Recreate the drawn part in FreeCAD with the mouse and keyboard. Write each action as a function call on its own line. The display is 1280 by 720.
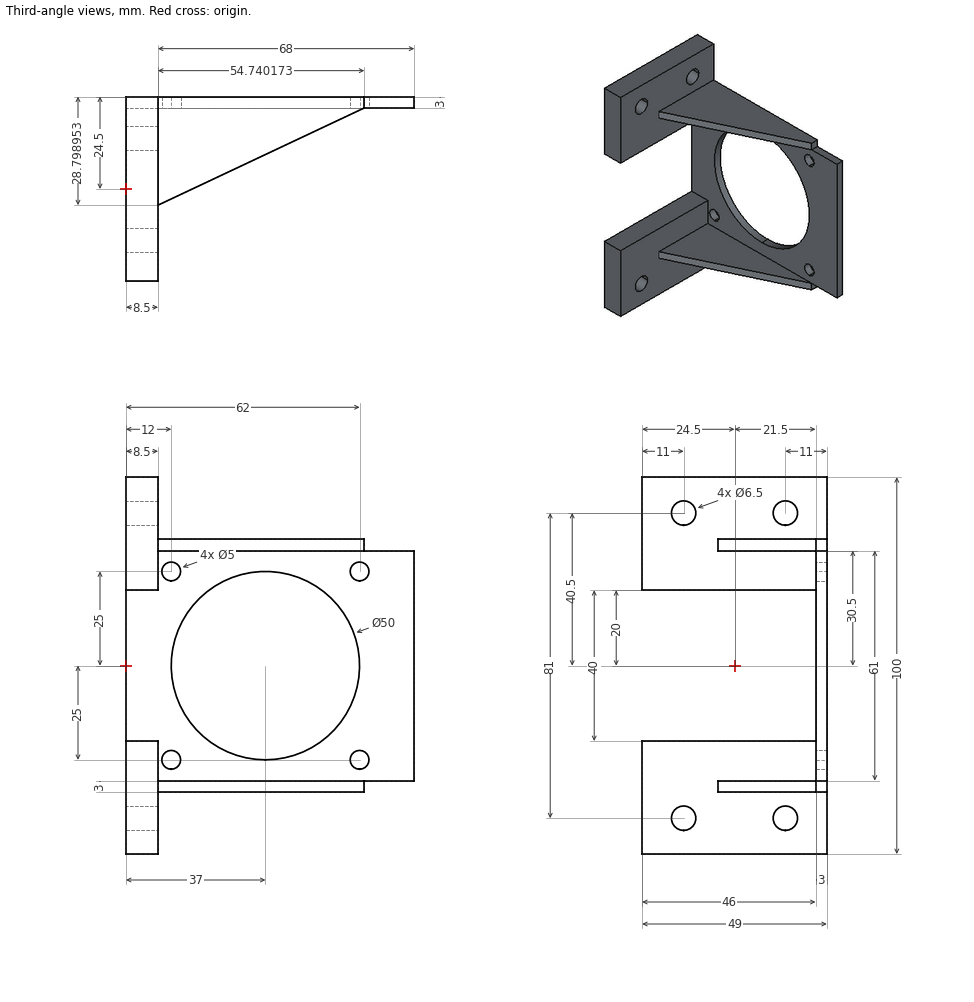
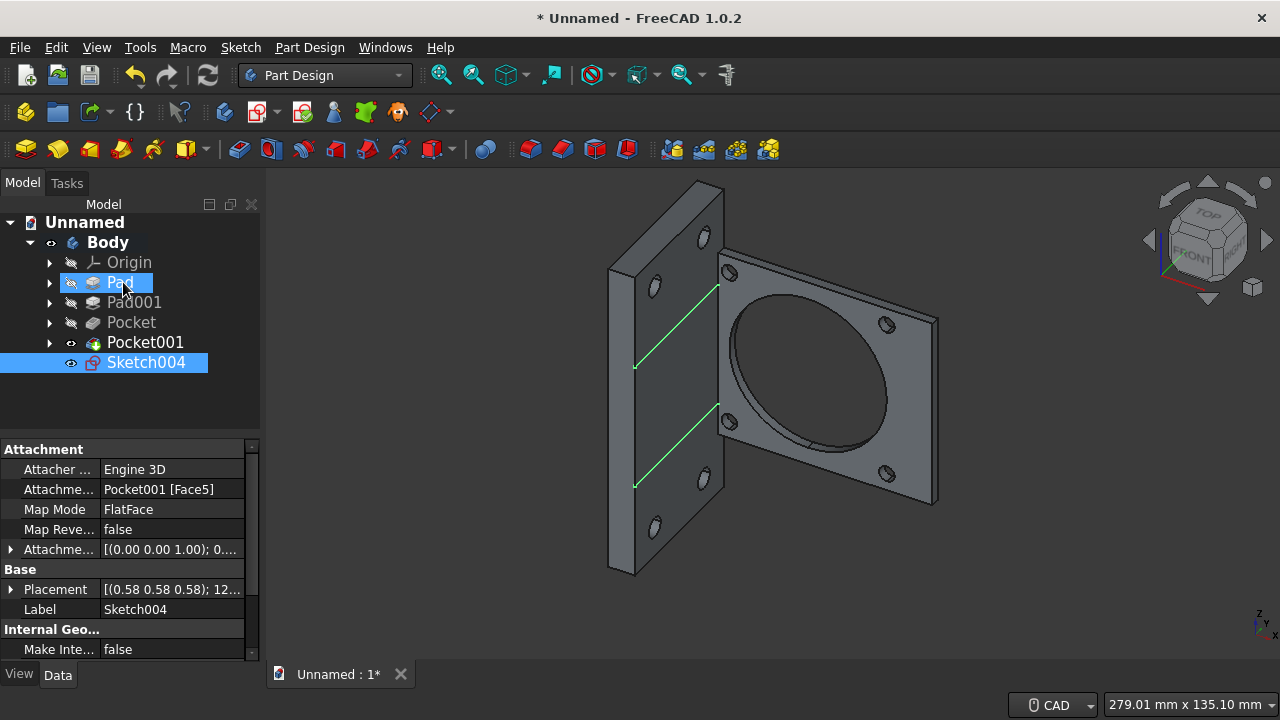
click(240, 150)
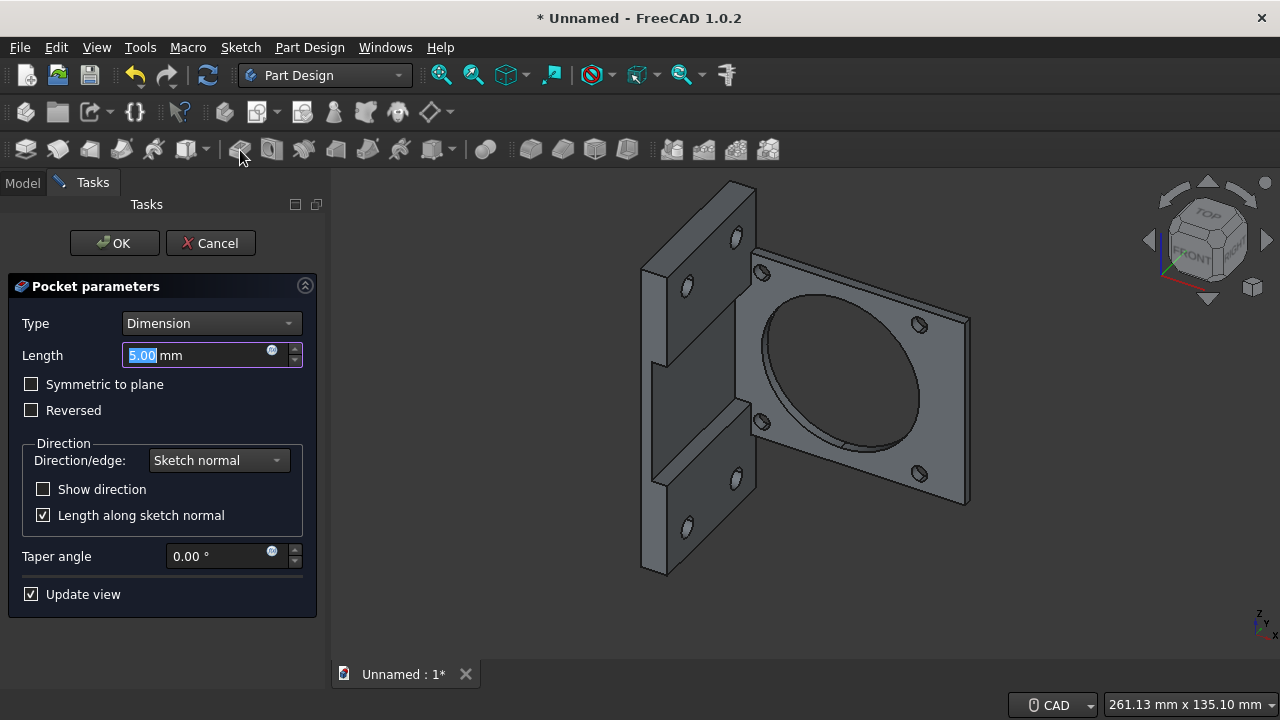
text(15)
key(Tab)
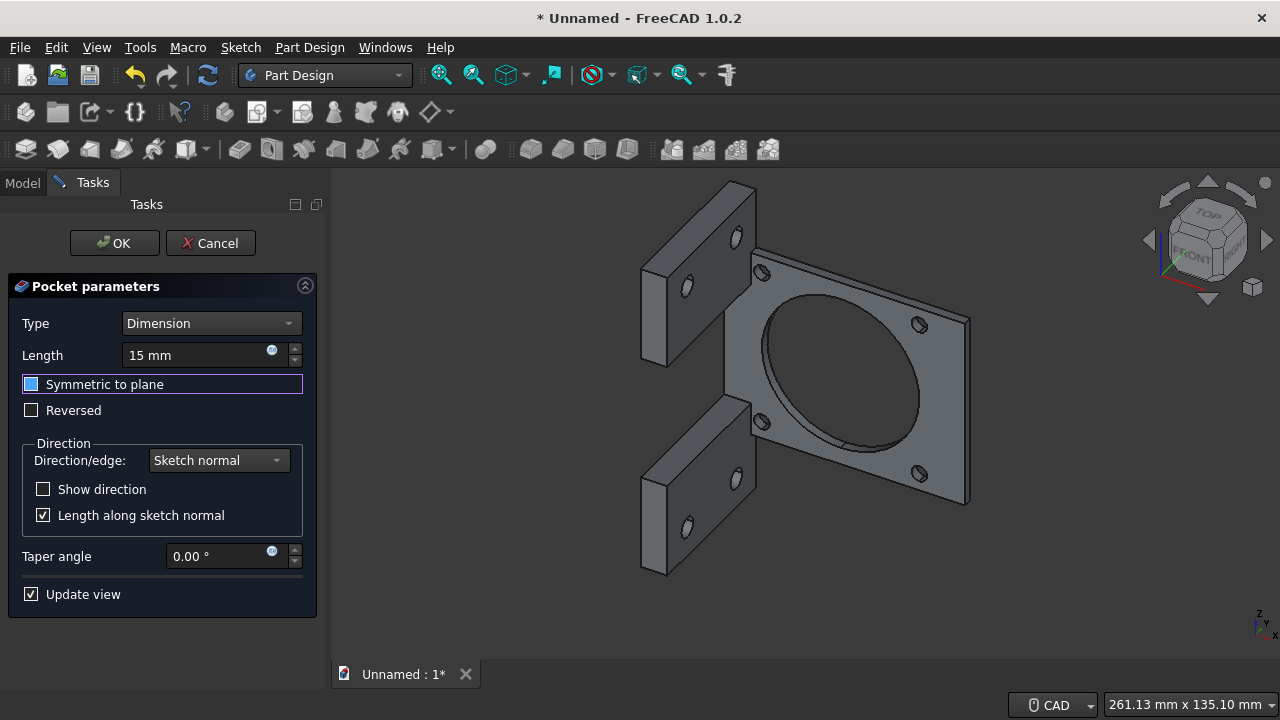
click(115, 243)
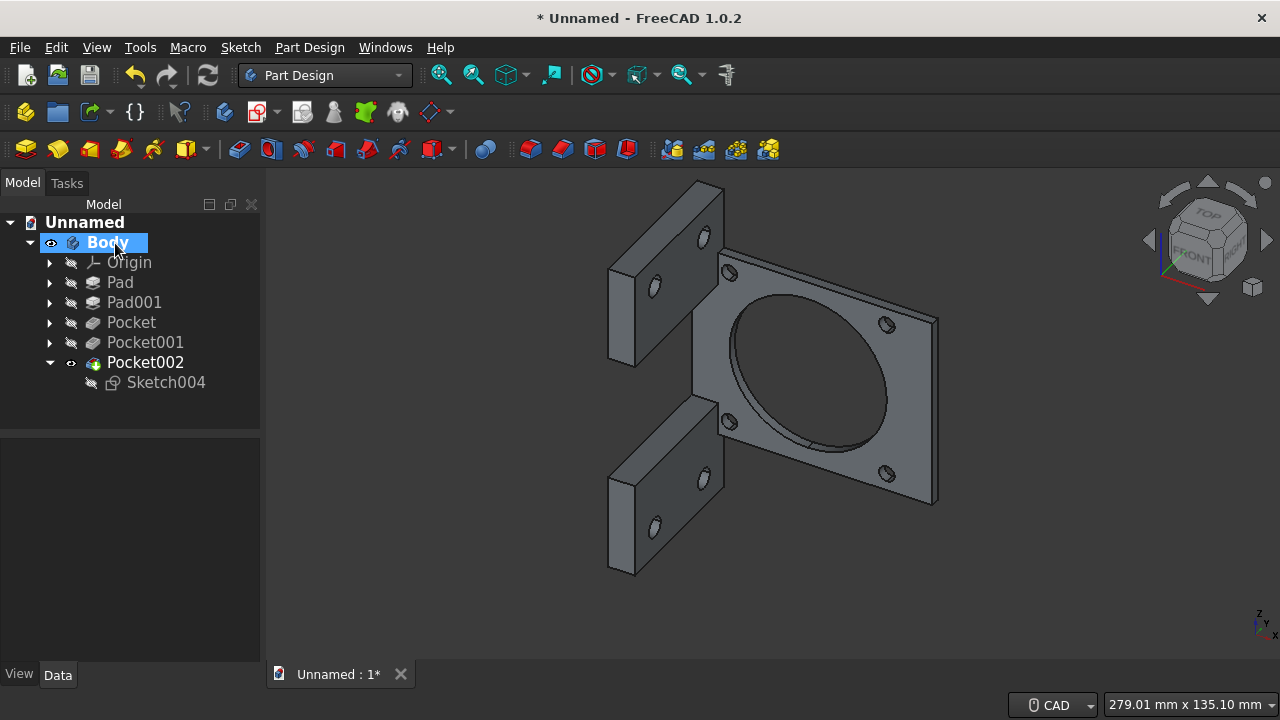
key(5)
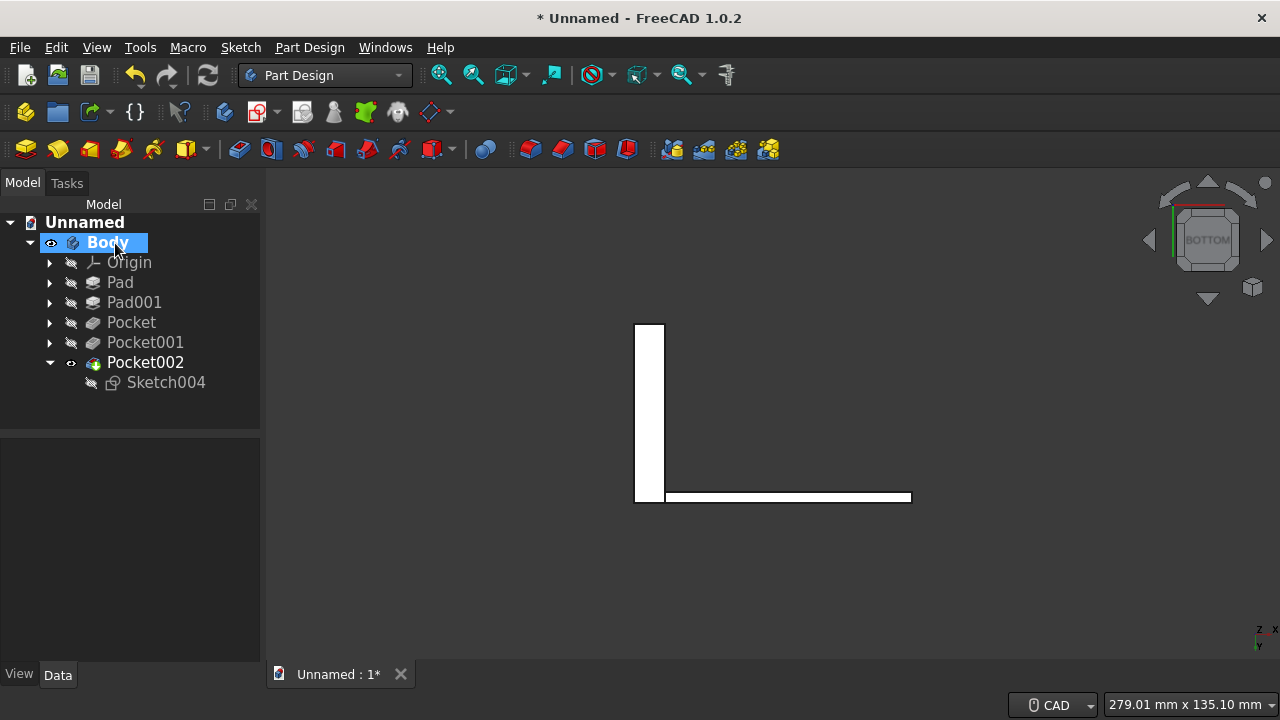
click(442, 76)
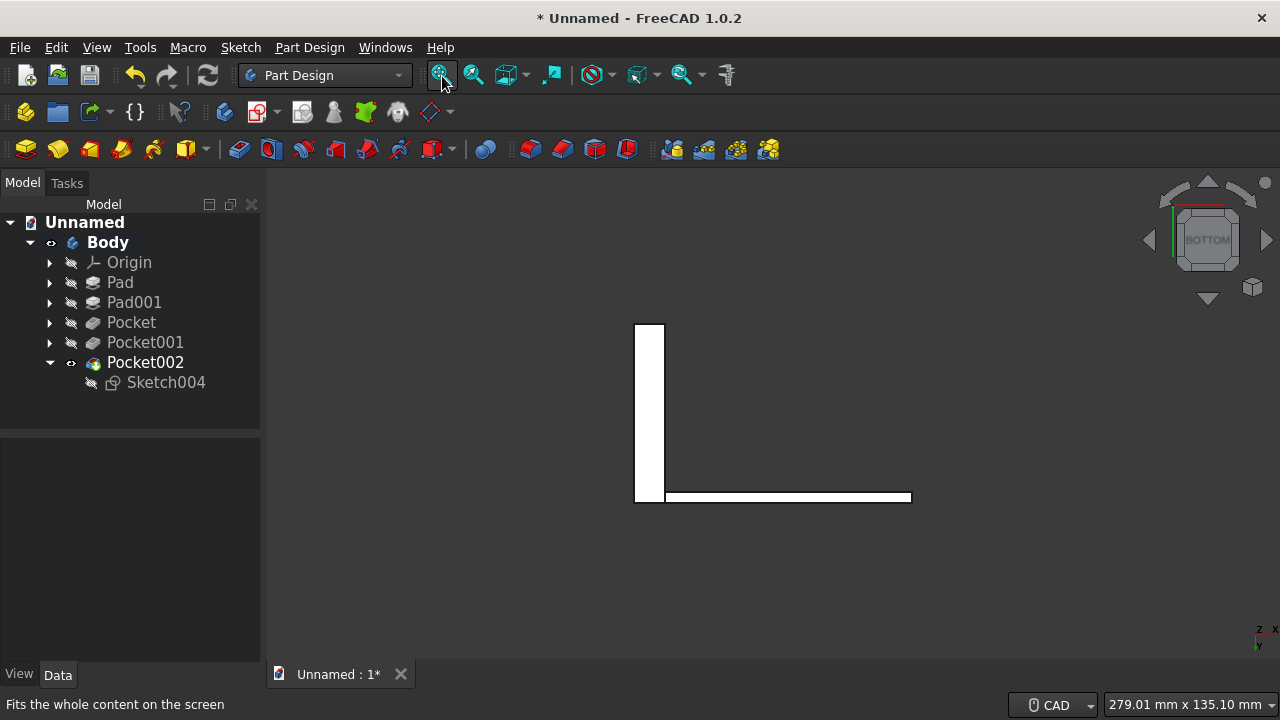
scroll(859, 496, up, 4)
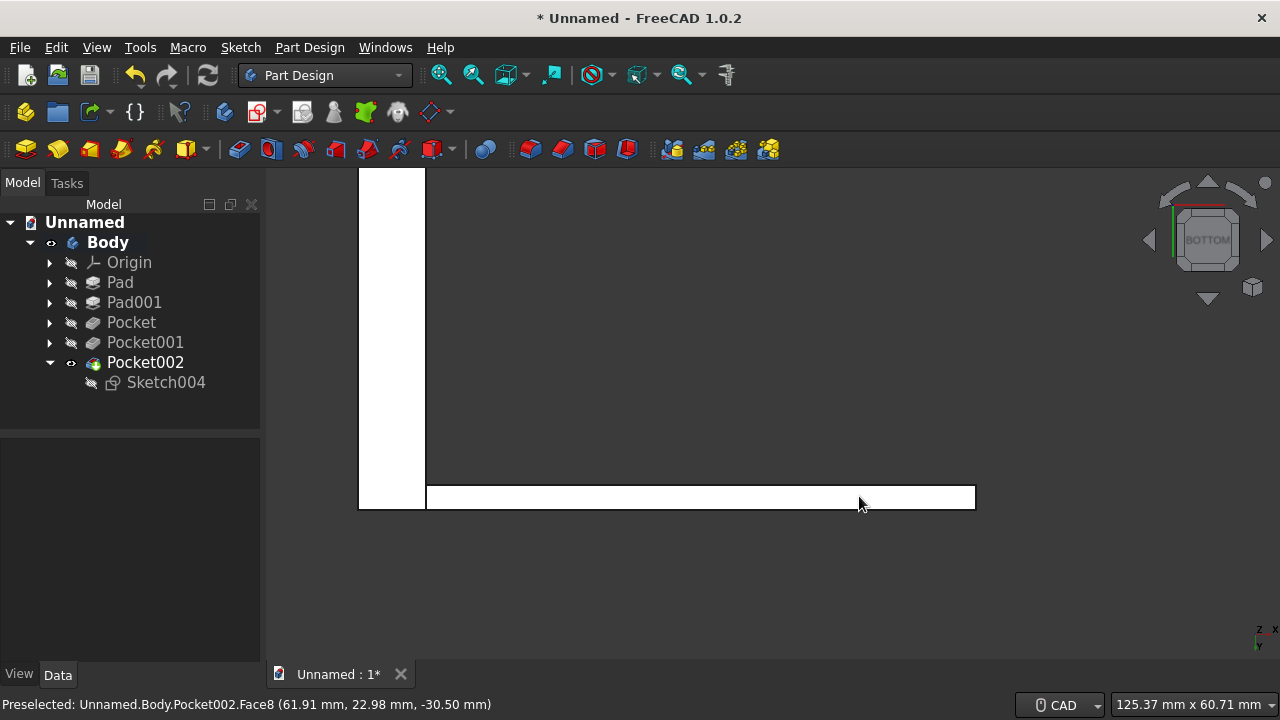
click(858, 497)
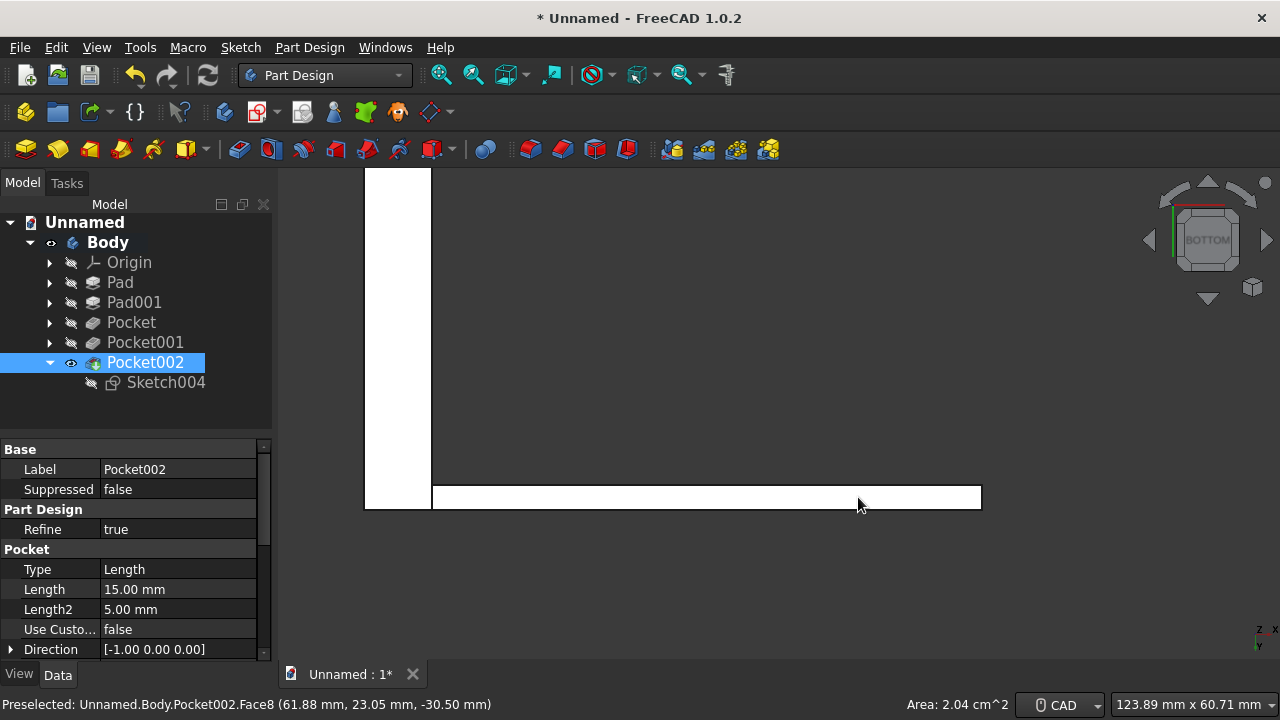
click(258, 112)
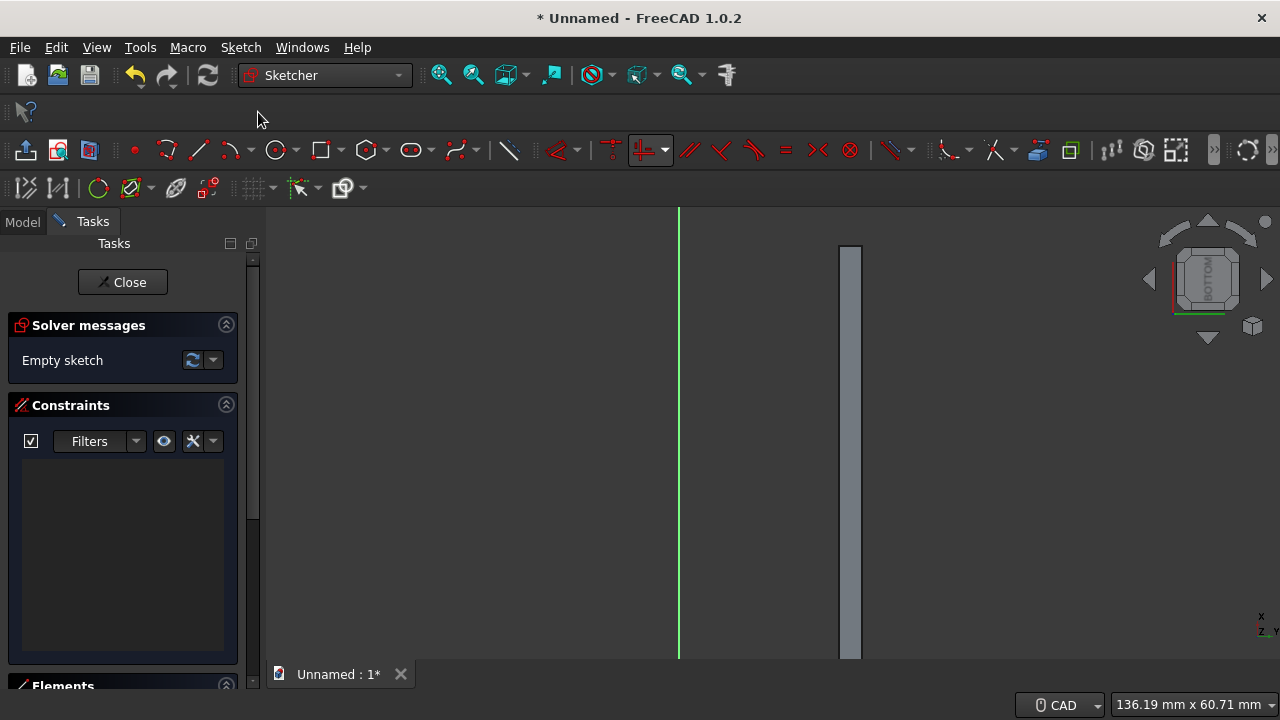
click(90, 150)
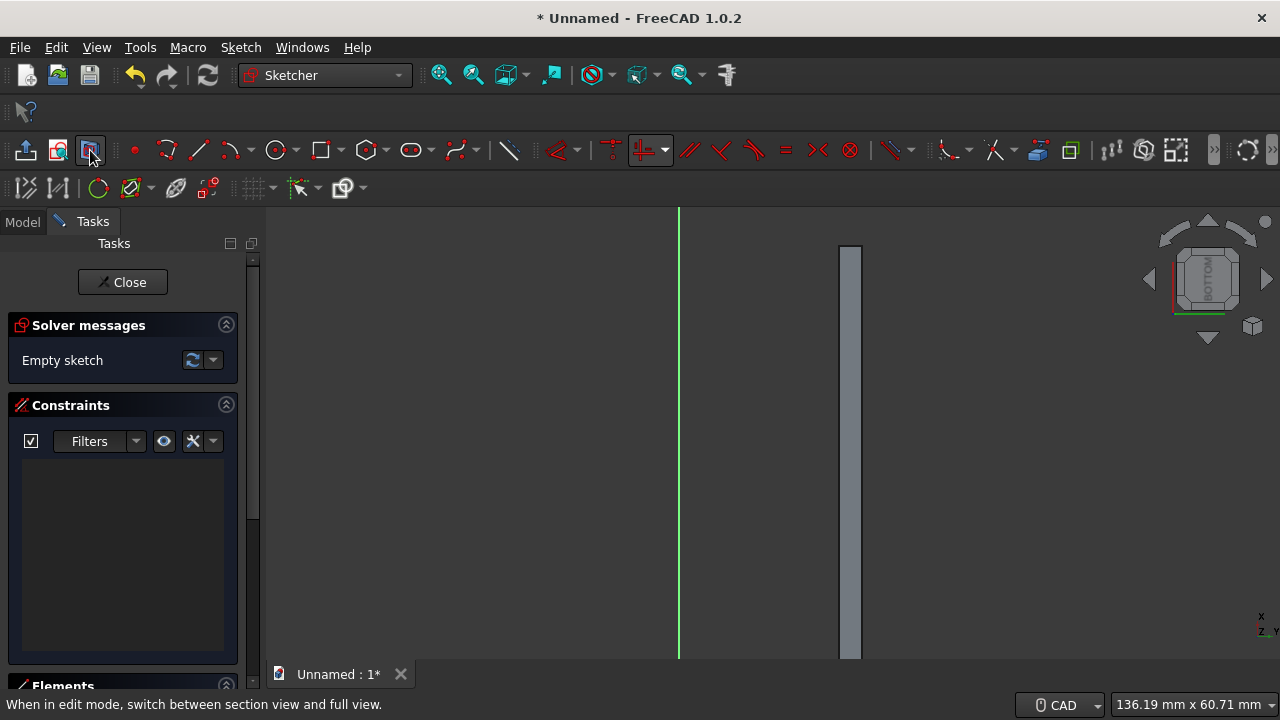
scroll(644, 254, down, 3)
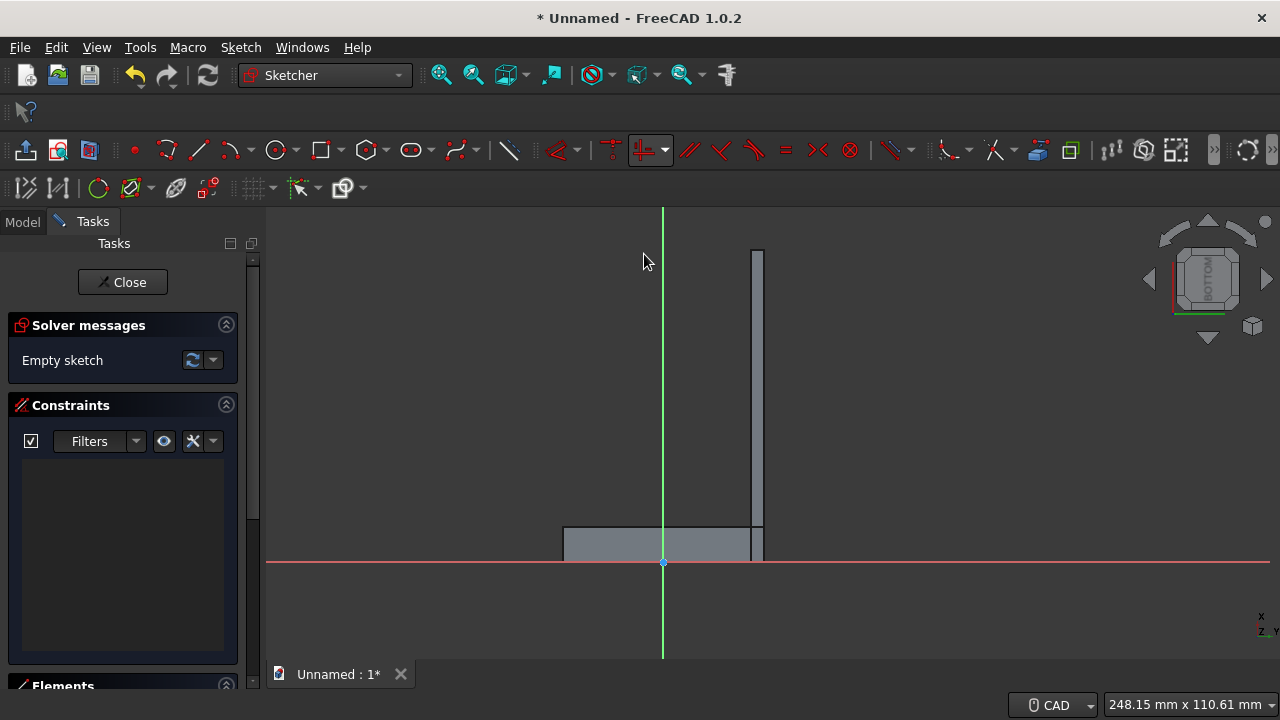
click(168, 150)